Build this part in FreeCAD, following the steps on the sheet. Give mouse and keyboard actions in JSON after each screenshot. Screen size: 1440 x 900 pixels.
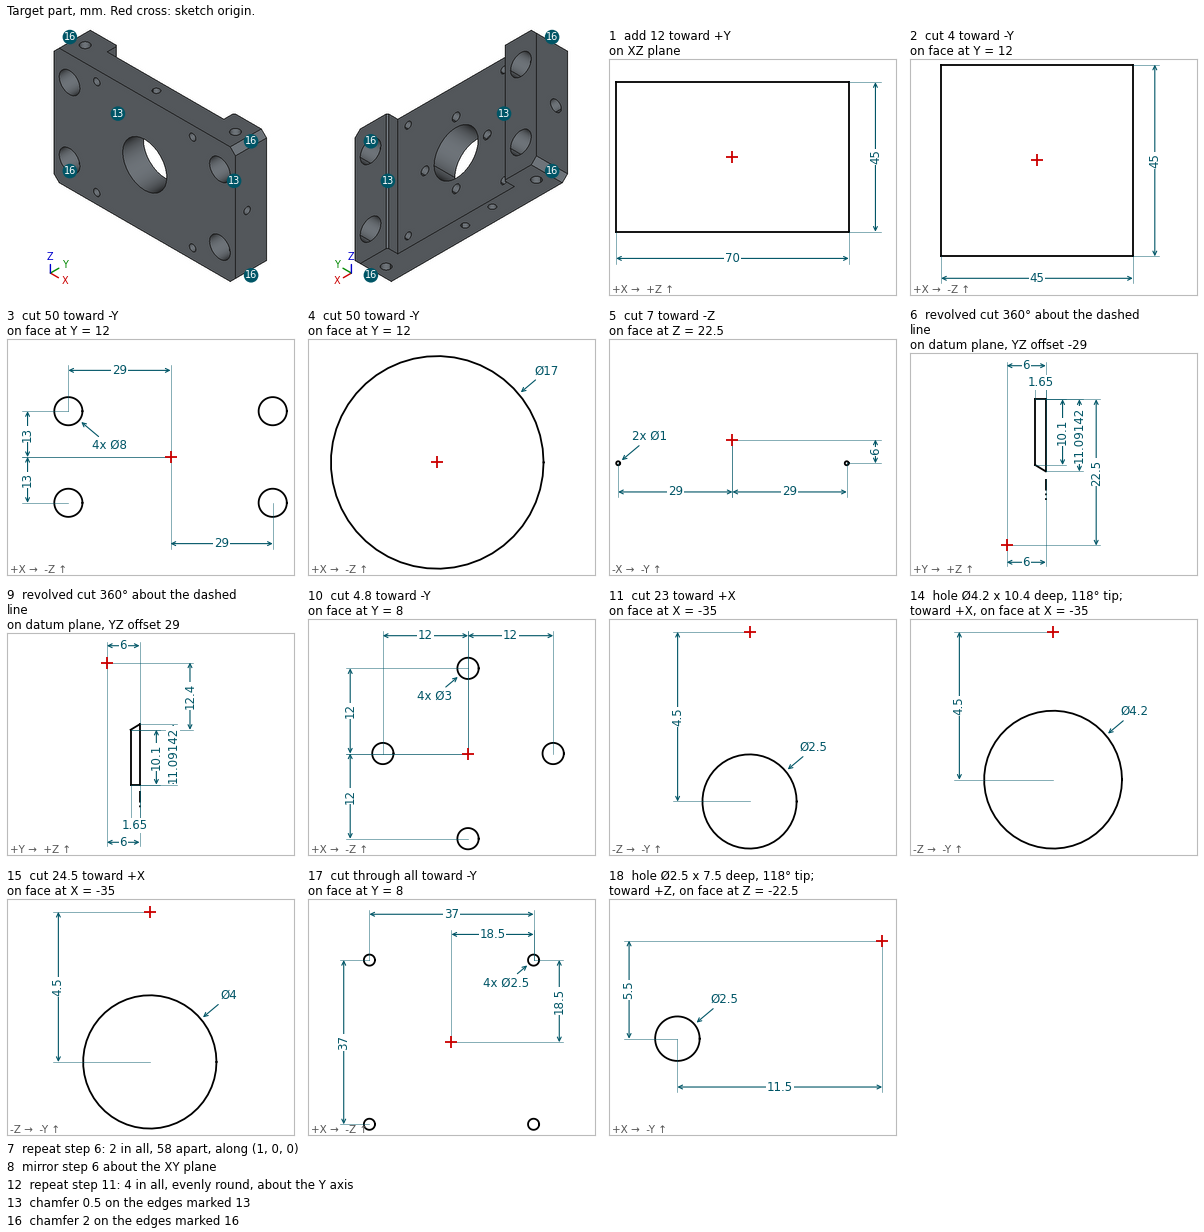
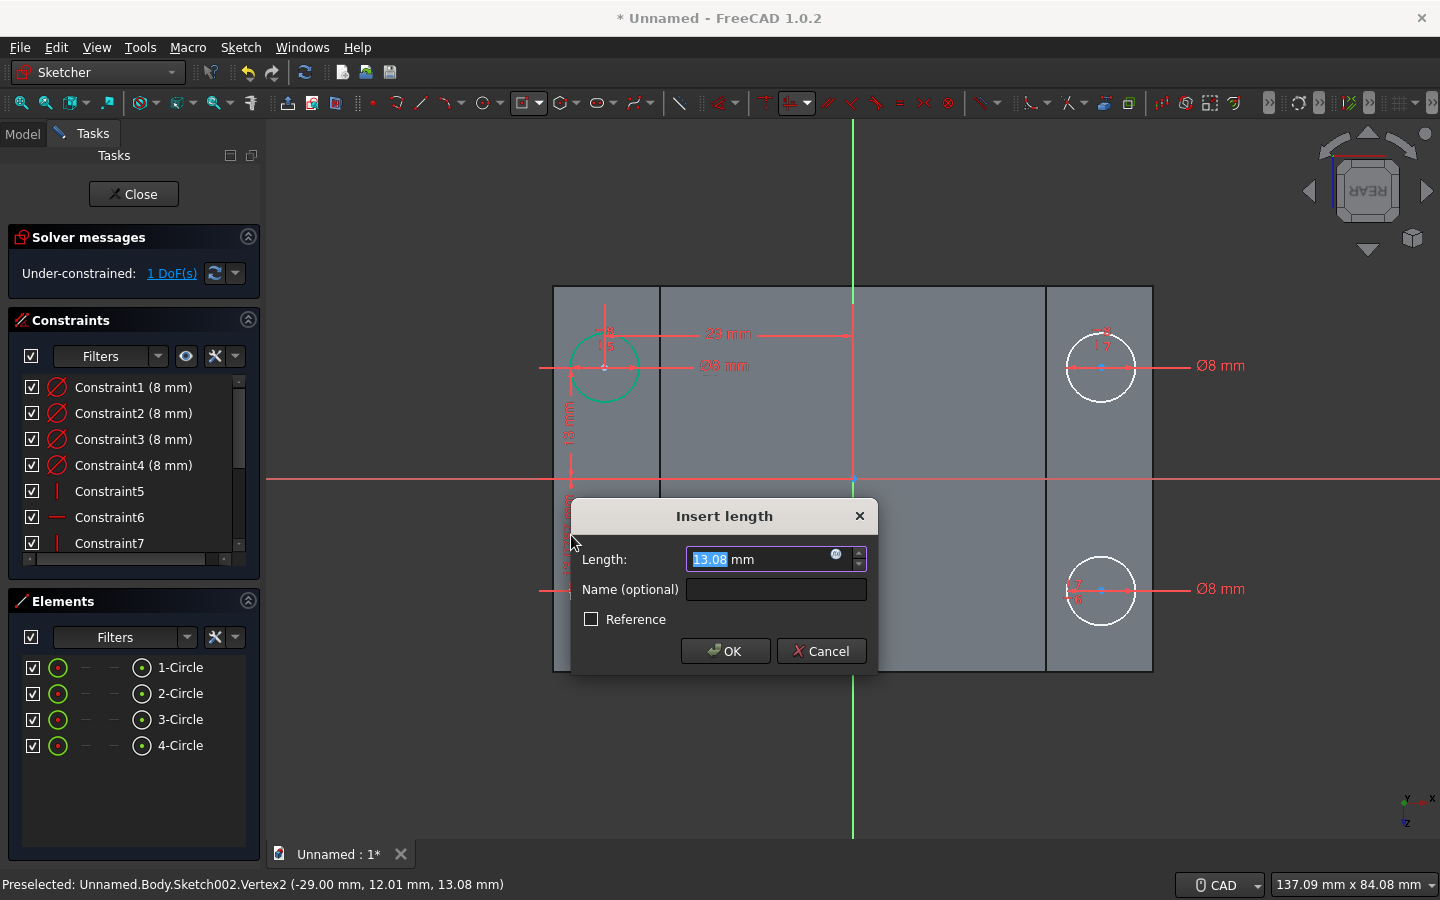
{"action": "type", "text": "13"}
{"action": "key", "text": "Return"}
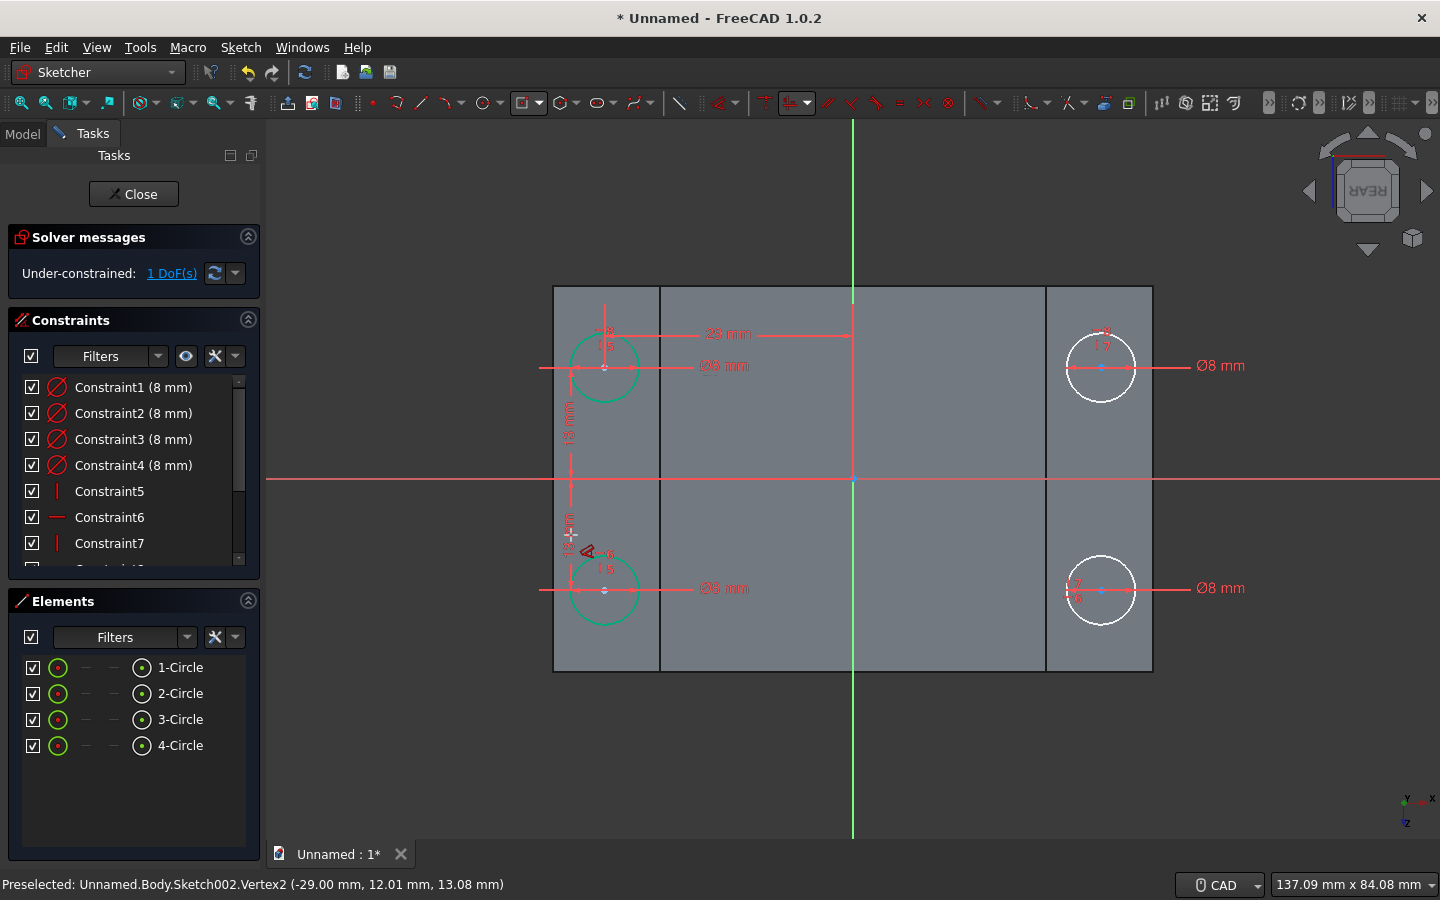
{"action": "left_click", "coordinate": [1101, 590]}
{"action": "left_click", "coordinate": [977, 624]}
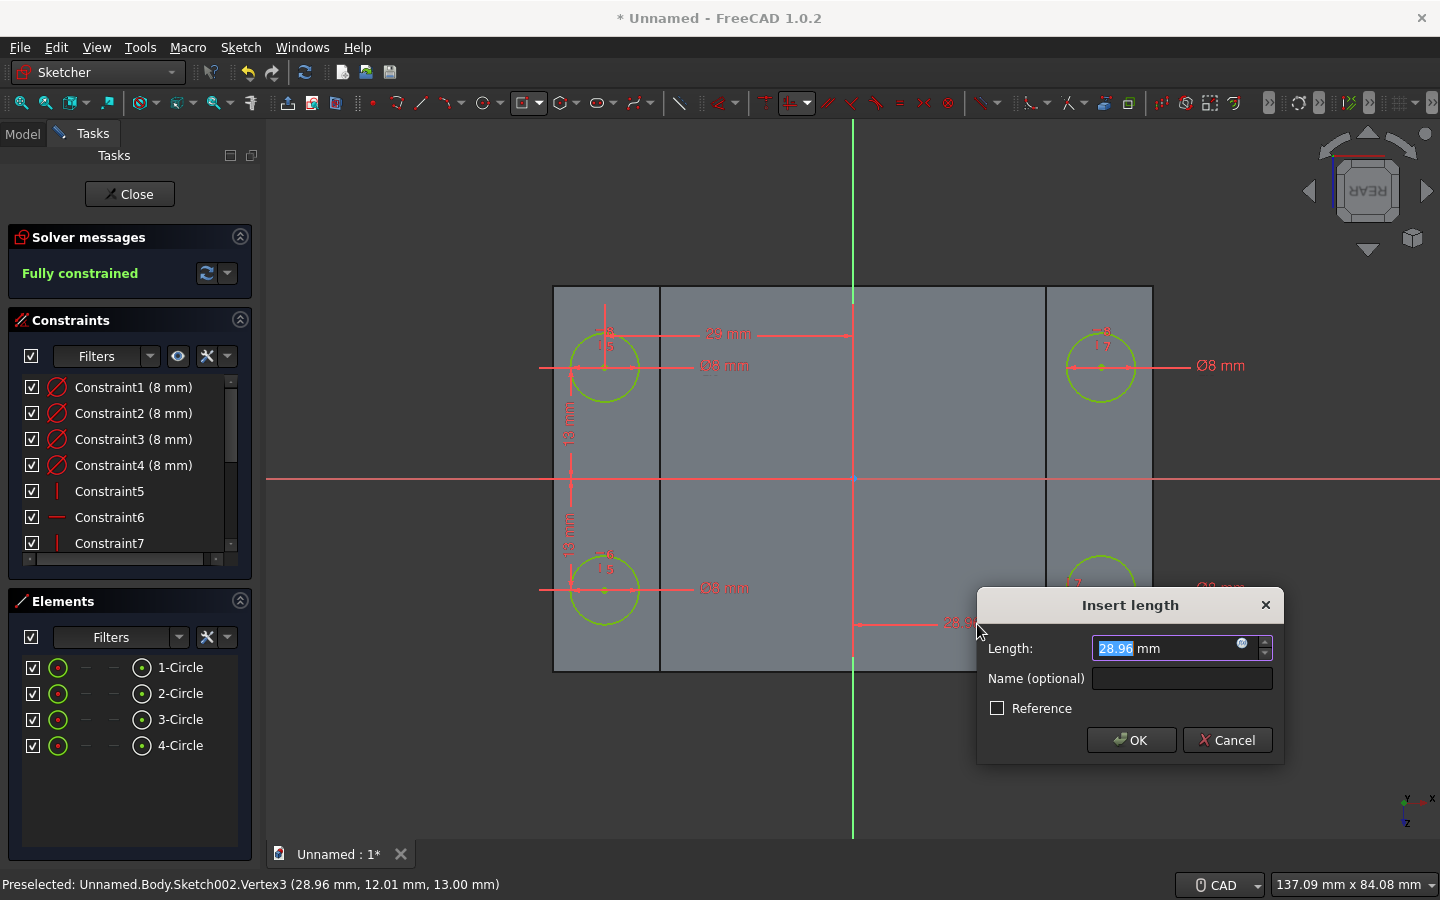
{"action": "type", "text": "29"}
{"action": "key", "text": "Return"}
{"action": "key", "text": "Escape"}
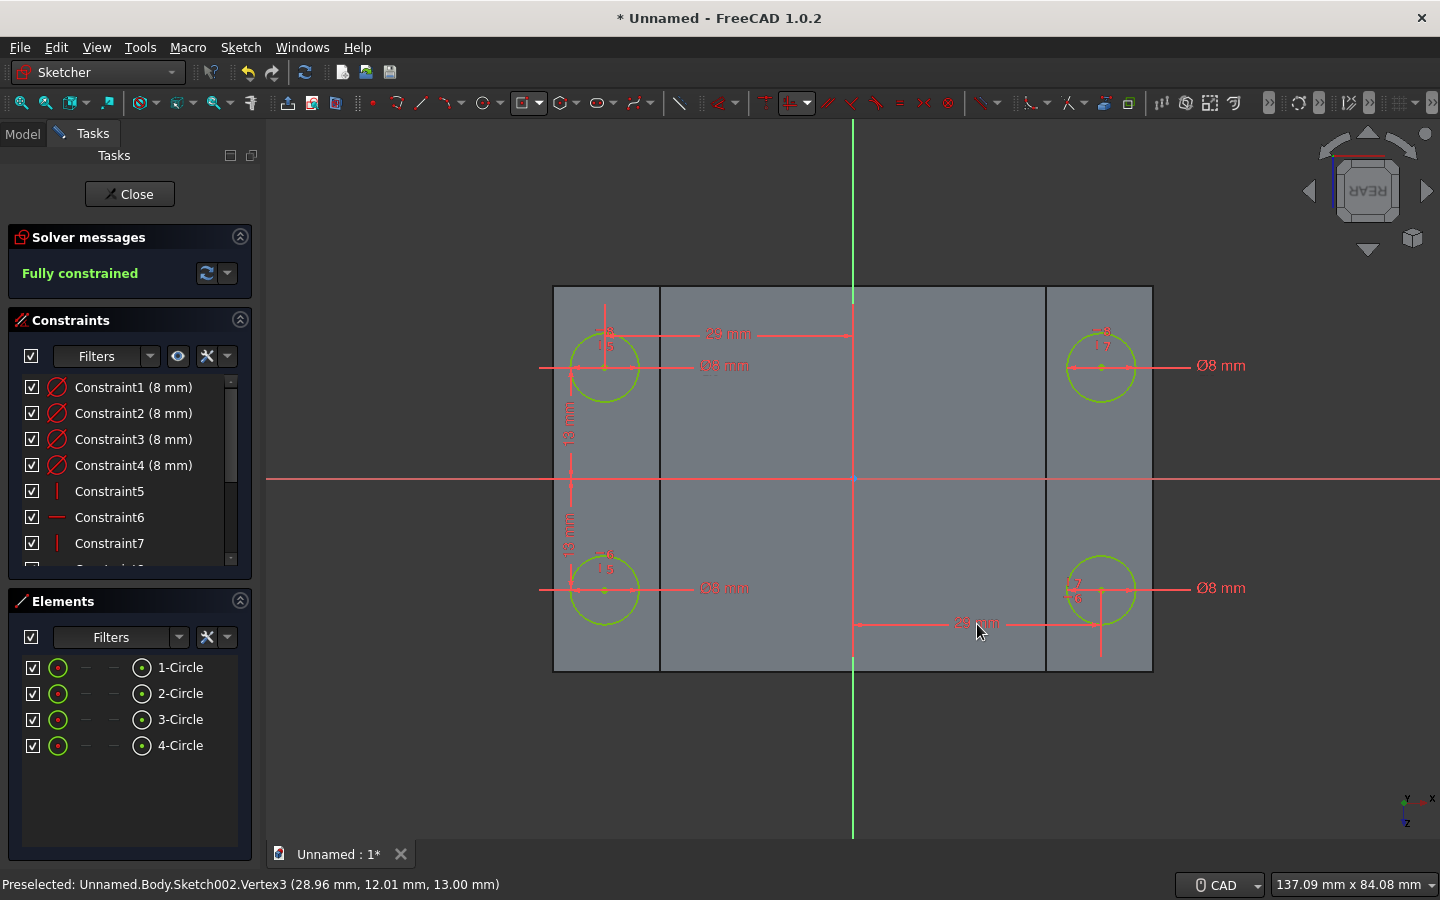
{"action": "left_click", "coordinate": [130, 194]}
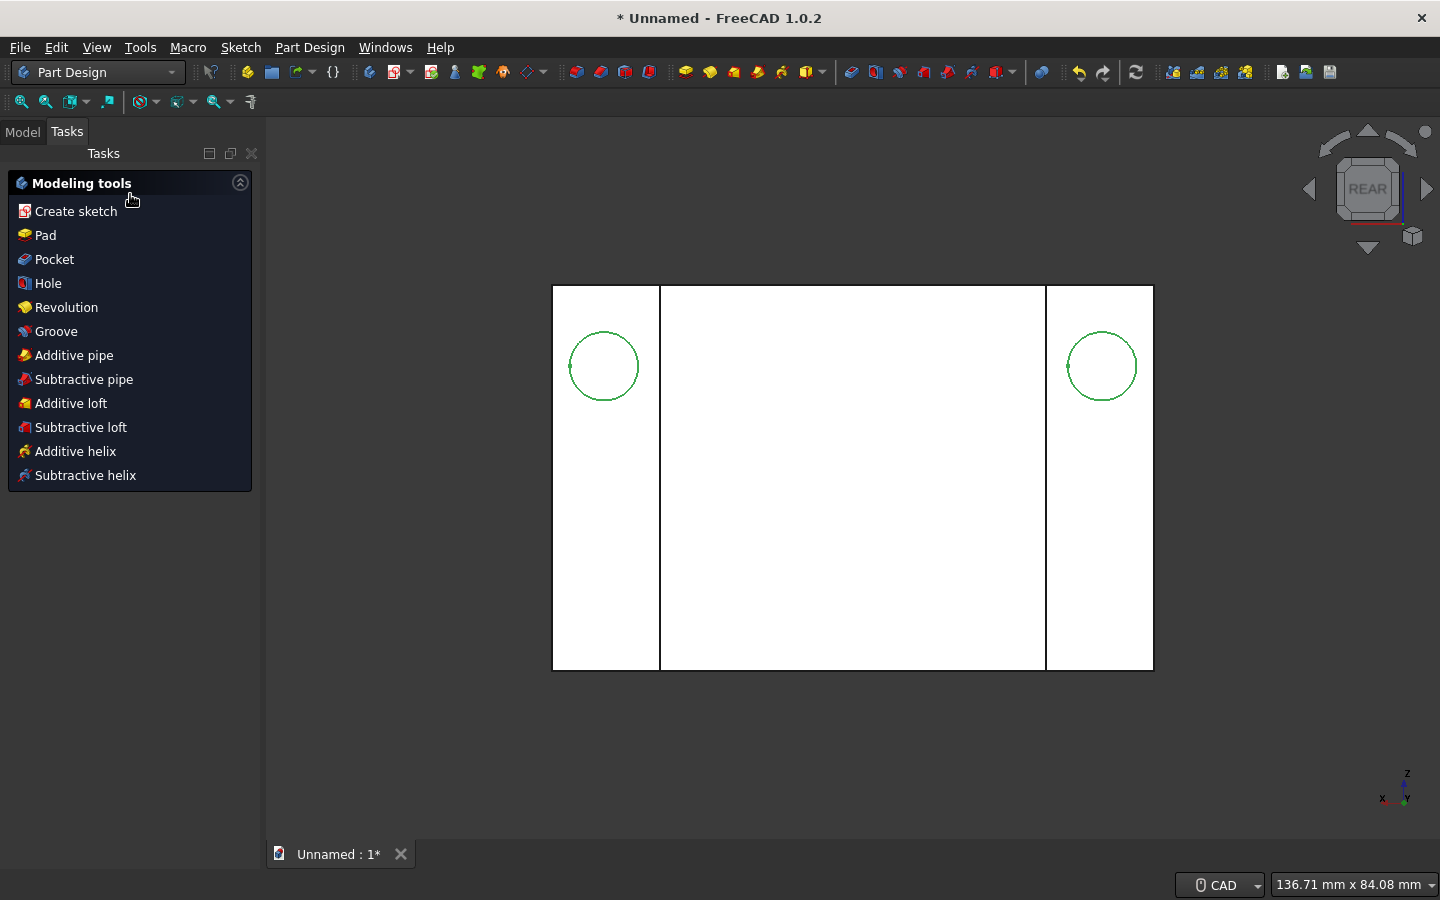
{"action": "left_click", "coordinate": [852, 72]}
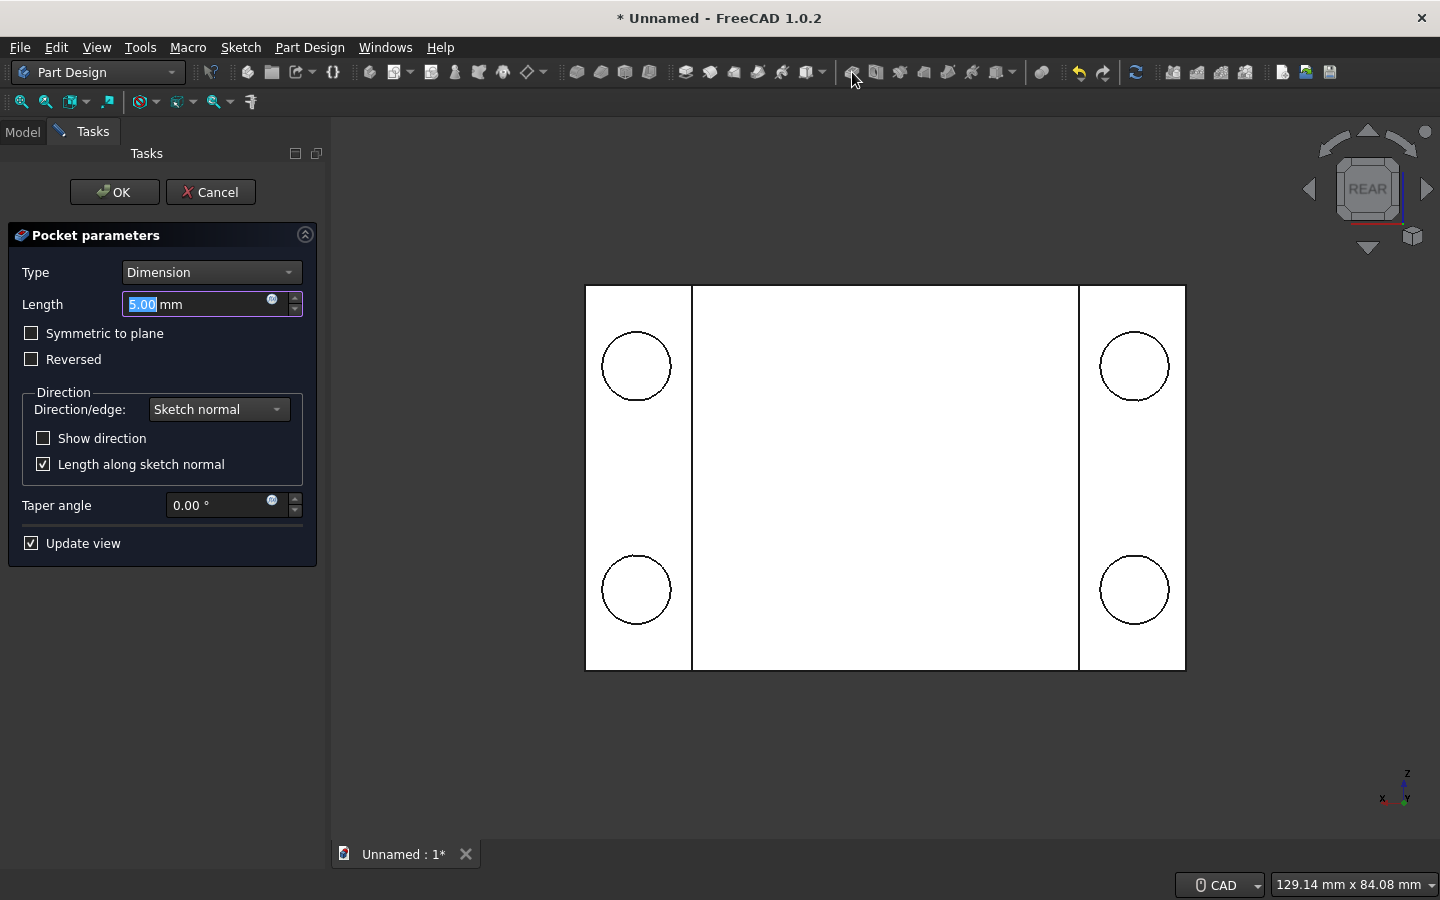
{"action": "type", "text": "50"}
{"action": "key", "text": "Tab"}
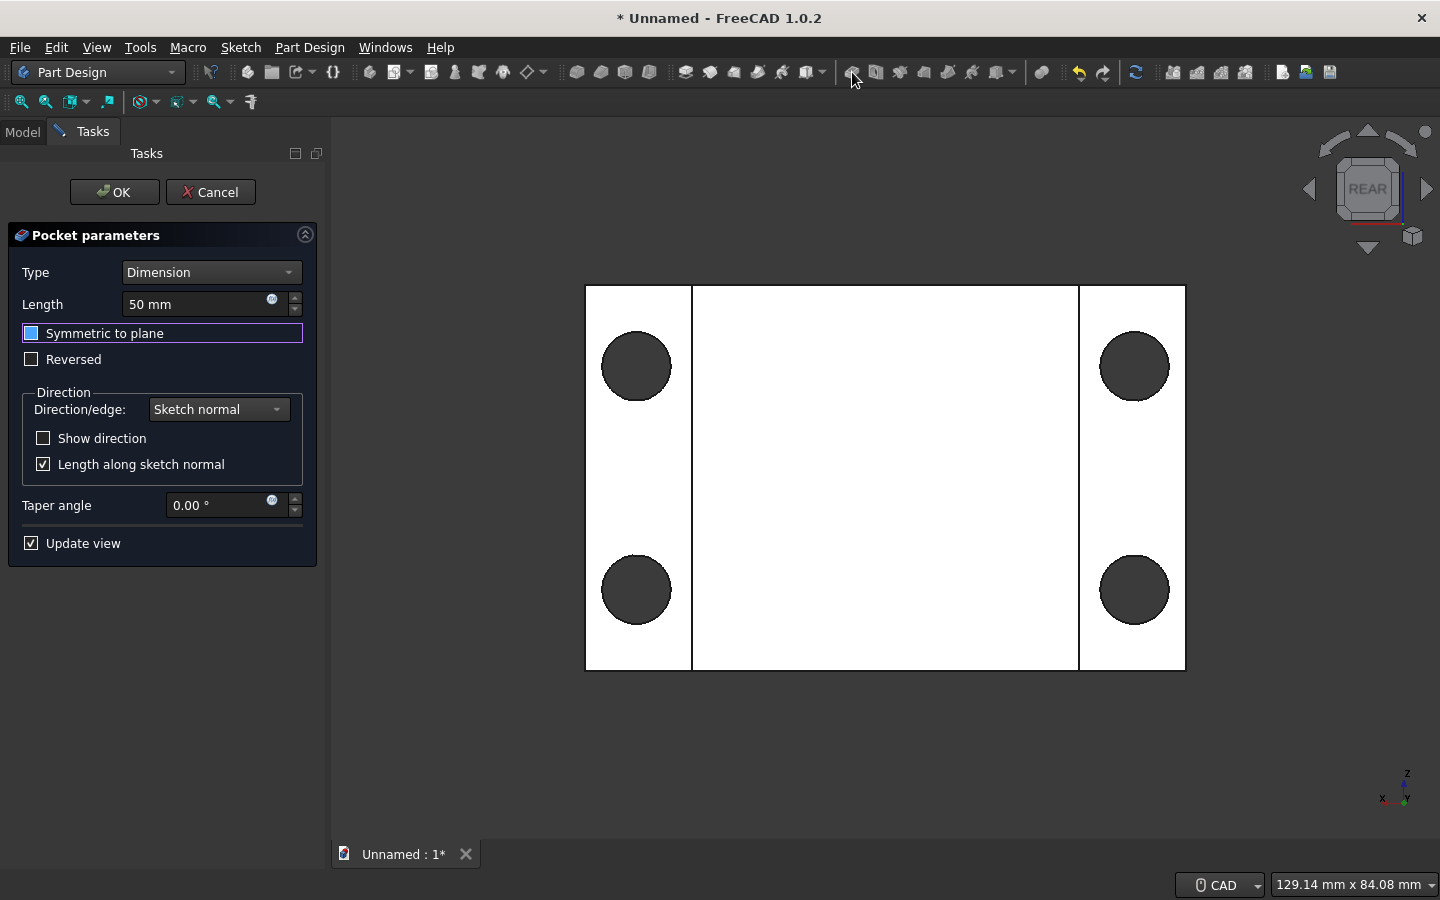
{"action": "left_click", "coordinate": [115, 192]}